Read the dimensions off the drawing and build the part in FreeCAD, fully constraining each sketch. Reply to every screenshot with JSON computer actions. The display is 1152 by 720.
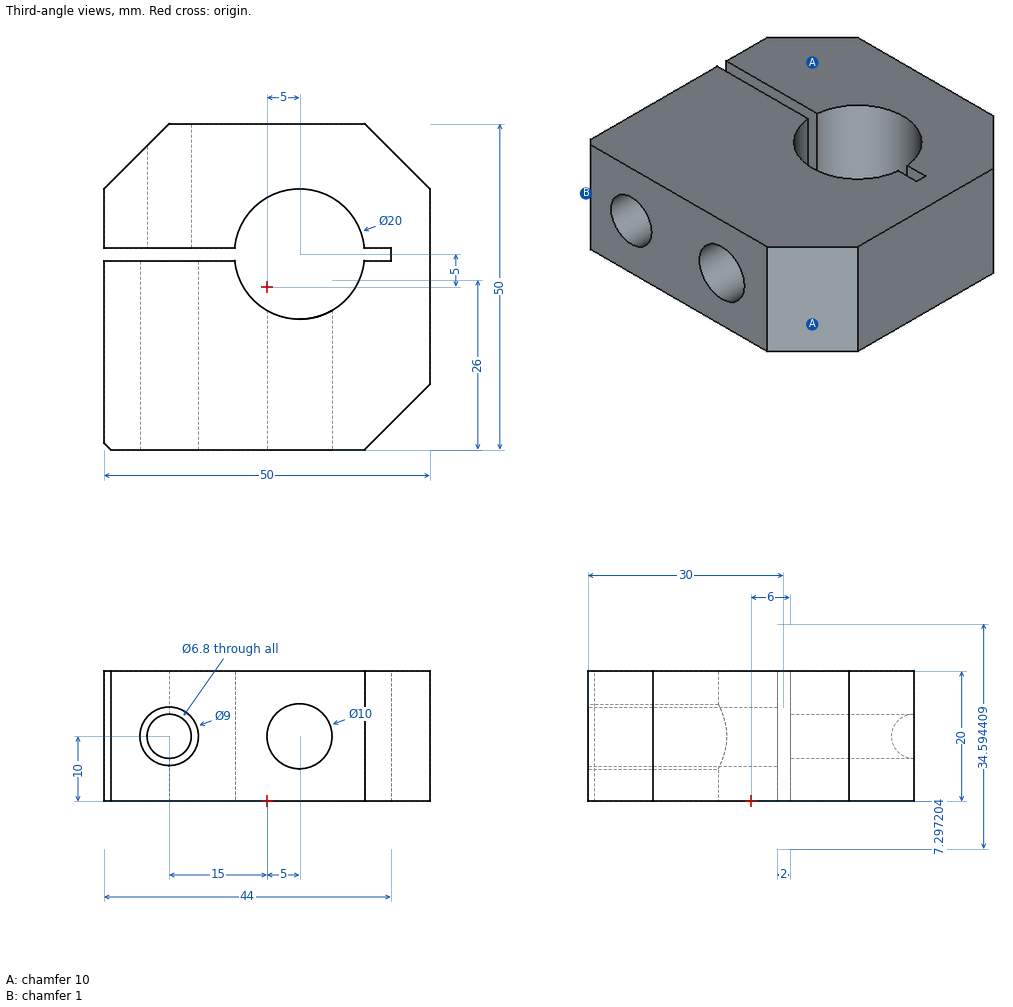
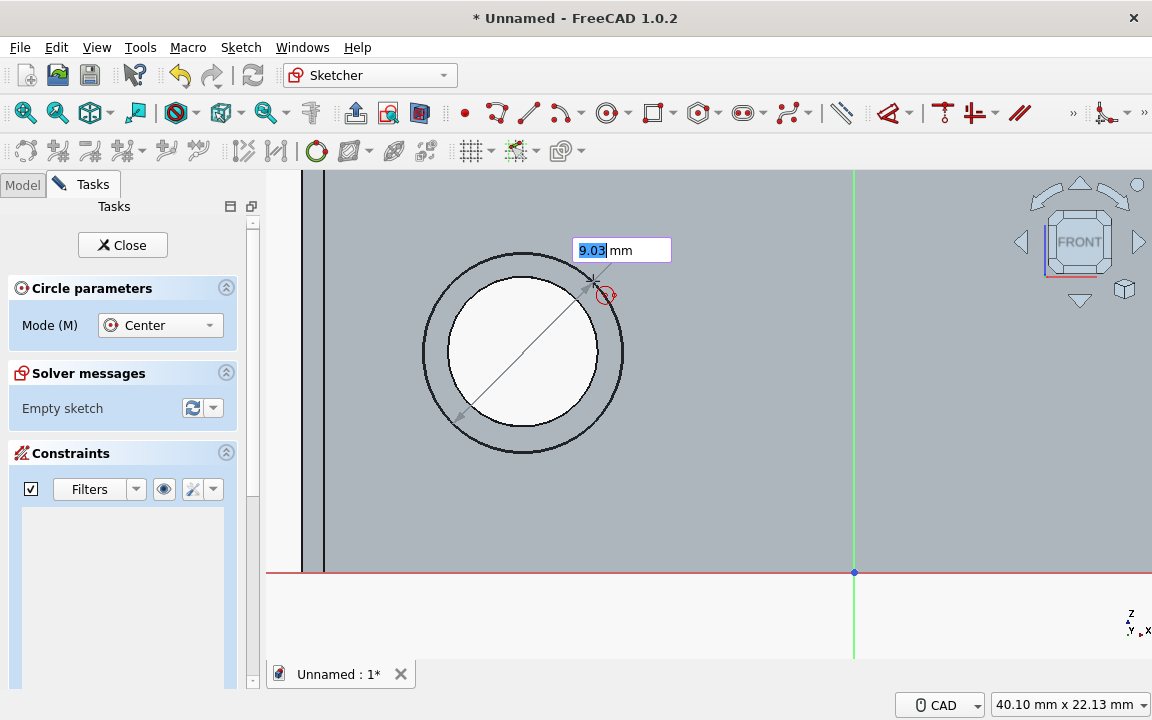
{"action": "type", "text": "9"}
{"action": "key", "text": "Return"}
{"action": "key", "text": "Escape"}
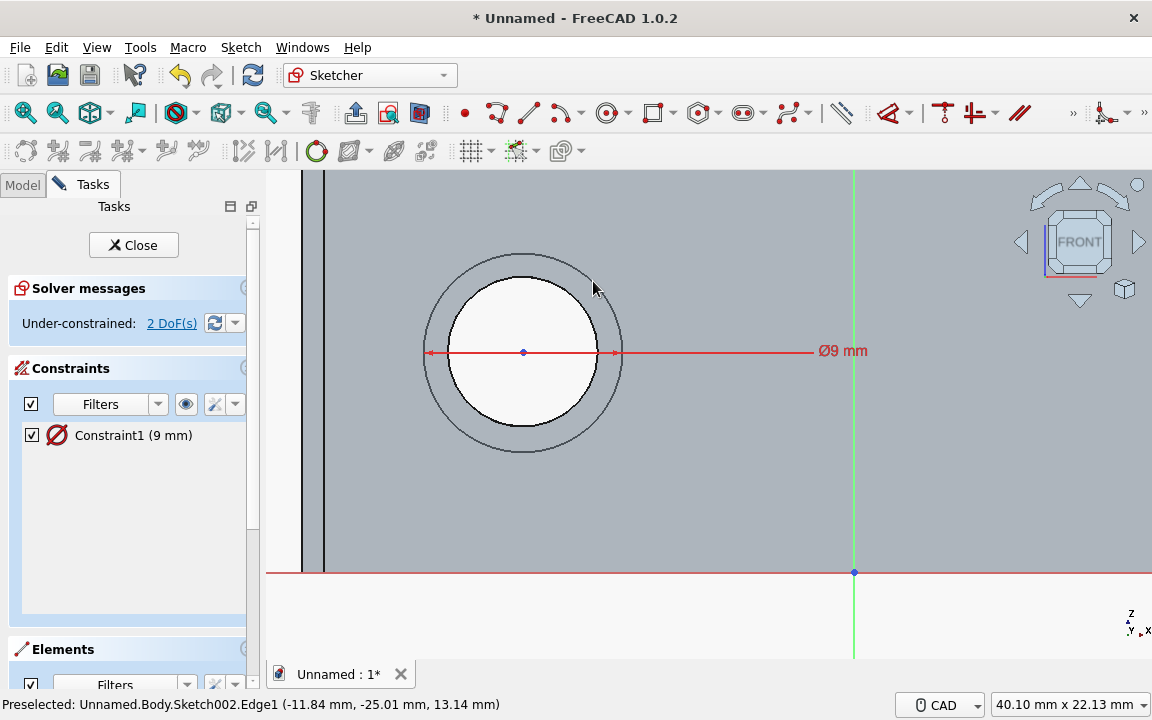
{"action": "left_click", "coordinate": [888, 114]}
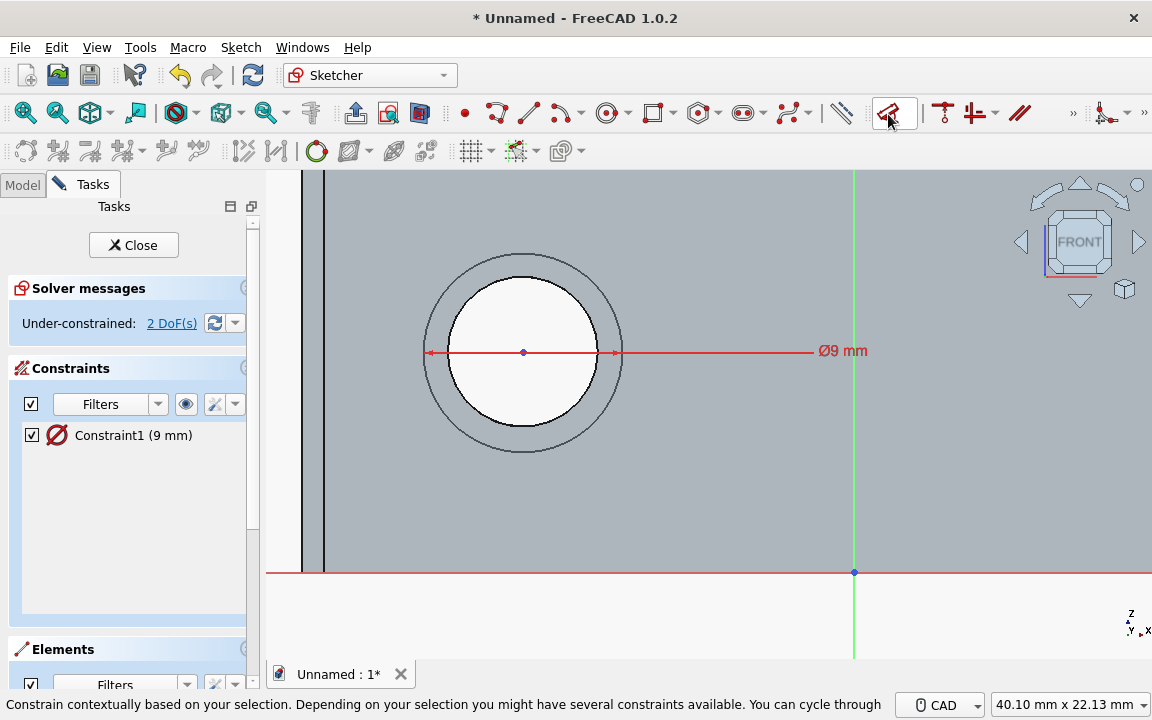
{"action": "left_click", "coordinate": [523, 353]}
{"action": "left_click", "coordinate": [689, 607]}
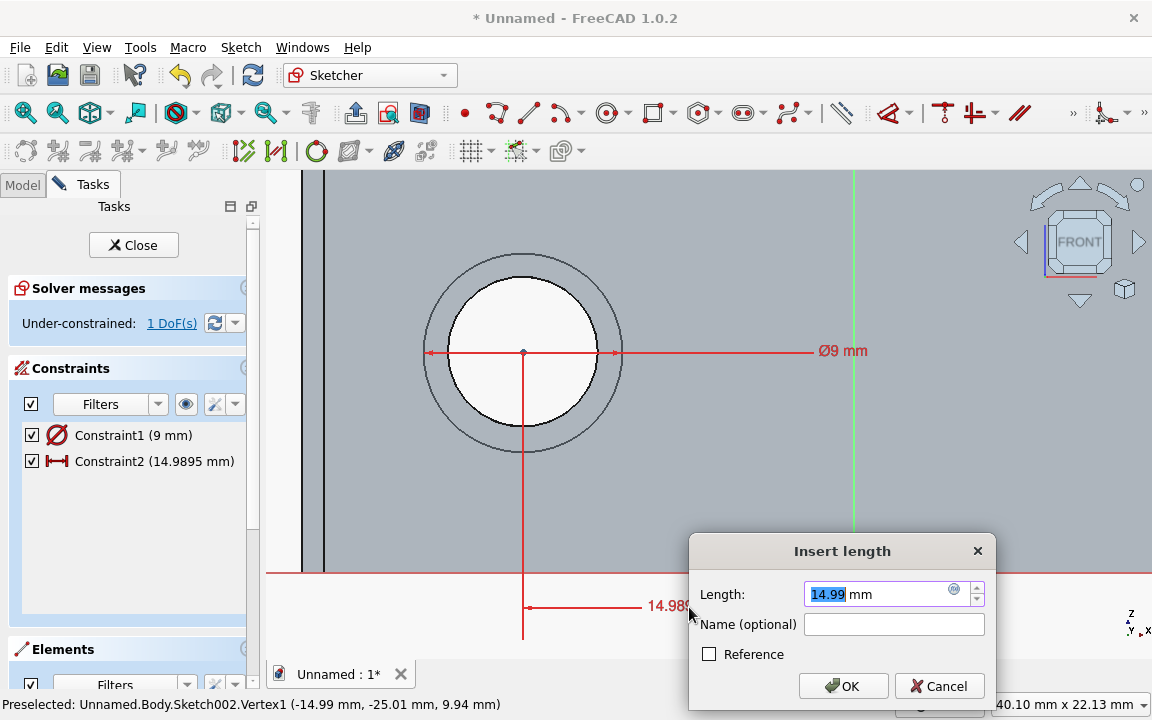
{"action": "type", "text": "15"}
{"action": "key", "text": "Return"}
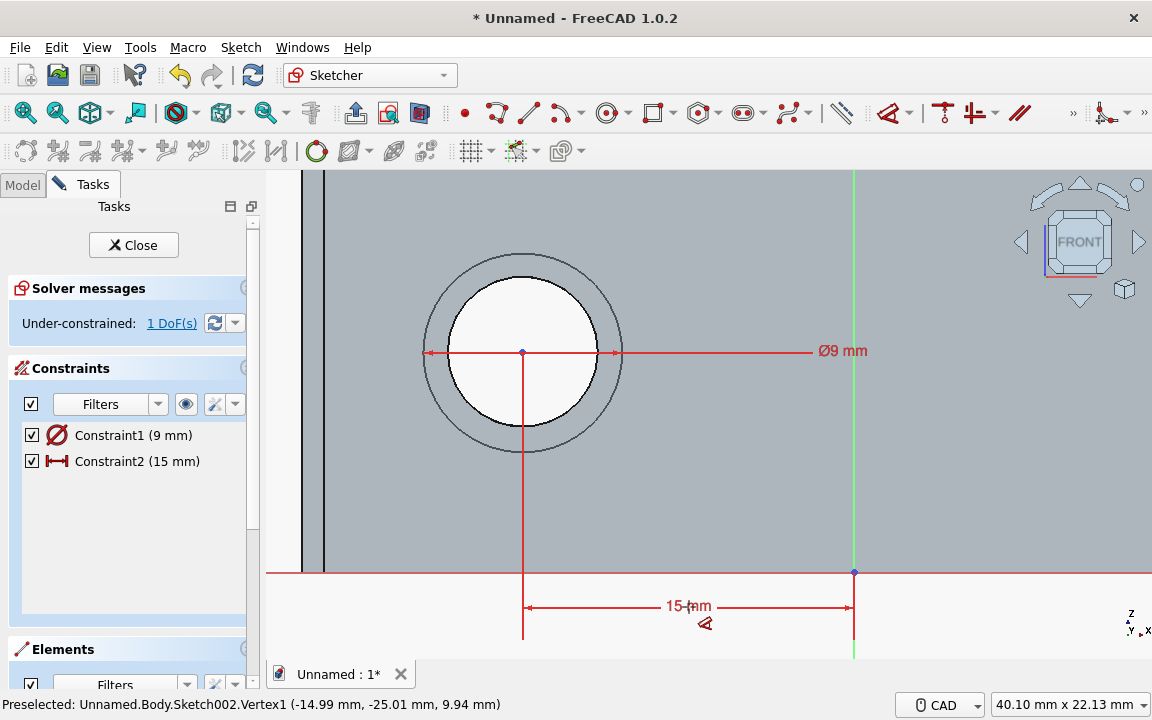
{"action": "left_click", "coordinate": [523, 353]}
{"action": "left_click", "coordinate": [888, 463]}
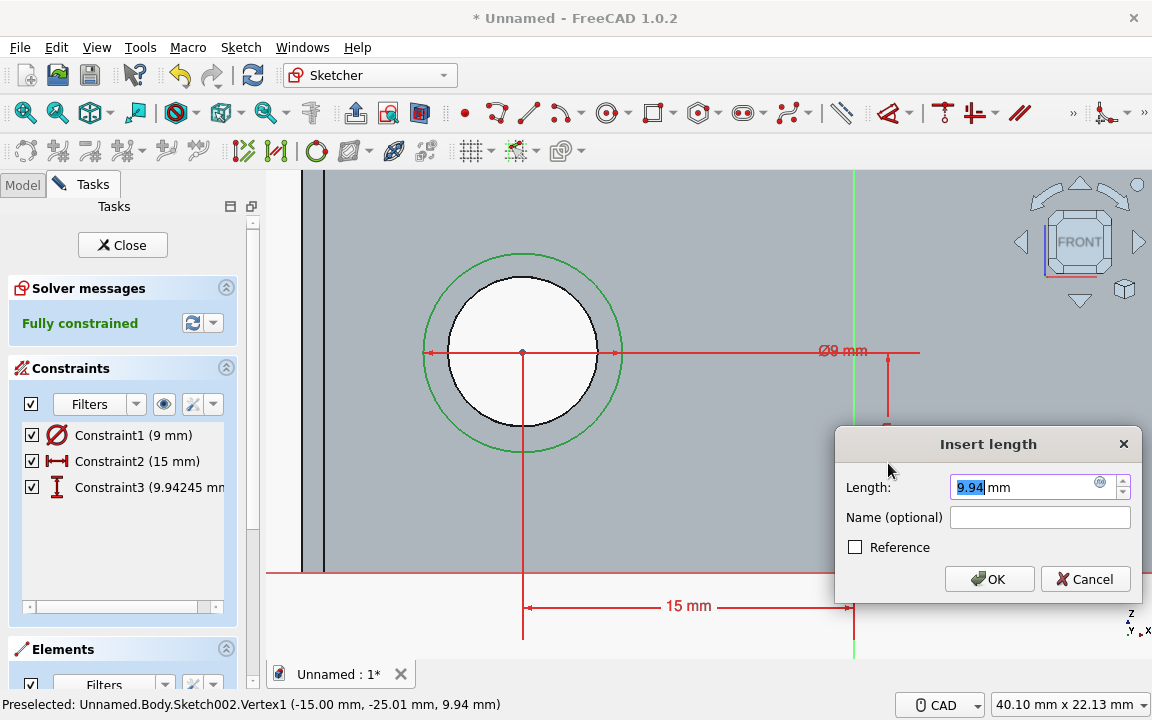
{"action": "type", "text": "10"}
{"action": "key", "text": "Return"}
{"action": "key", "text": "Escape"}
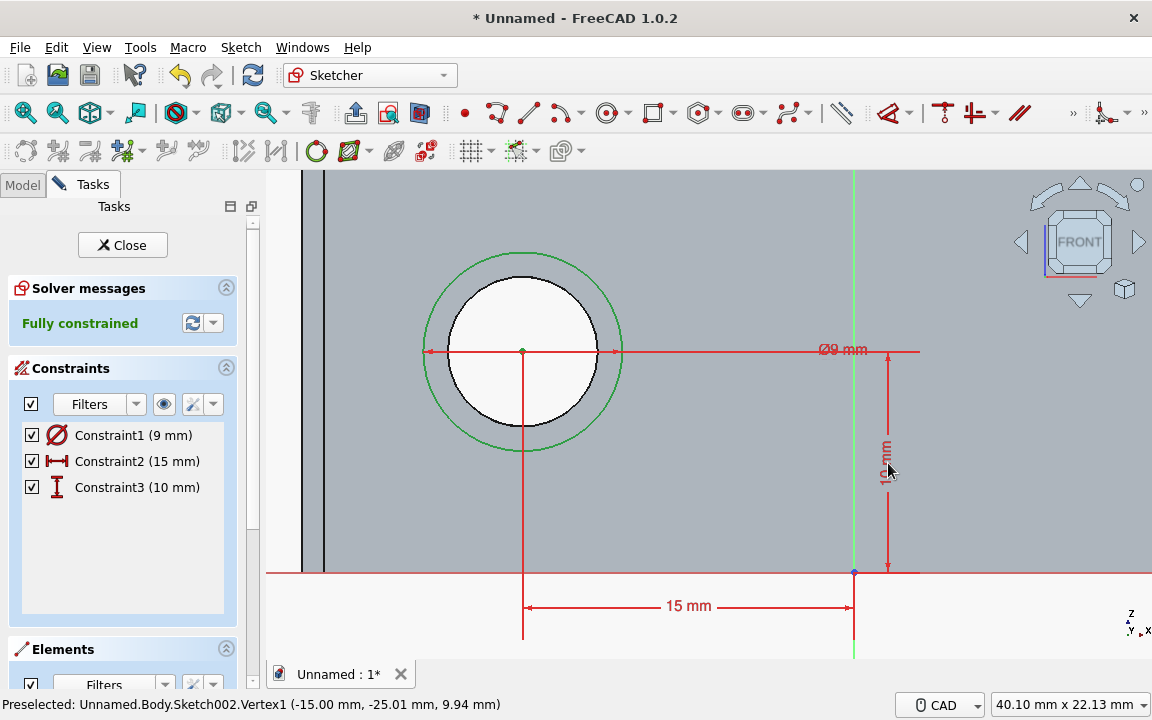
{"action": "left_click", "coordinate": [123, 245]}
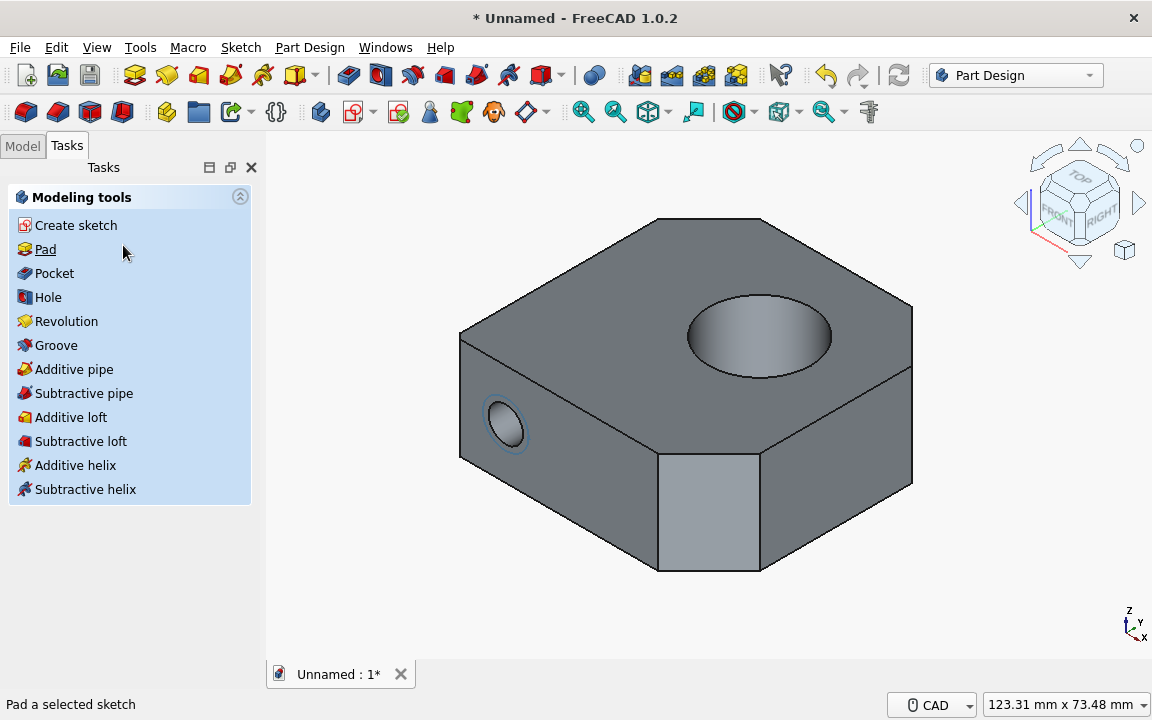
{"action": "left_click", "coordinate": [350, 76]}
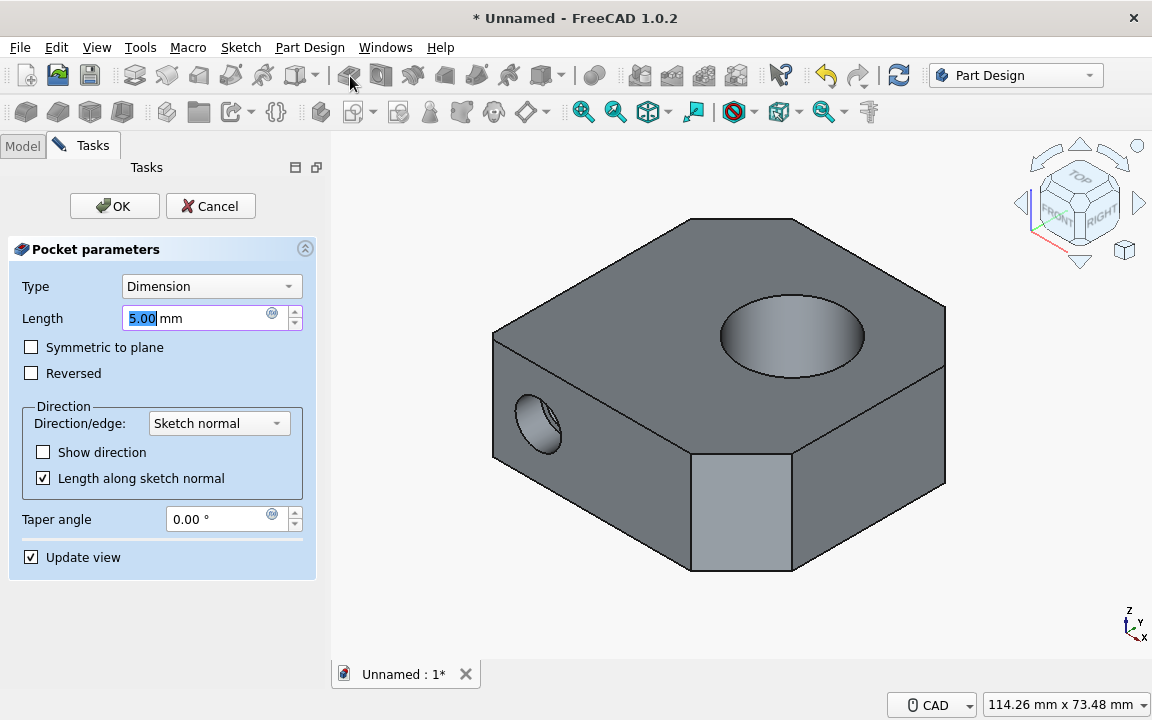
{"action": "type", "text": "30"}
{"action": "key", "text": "Tab"}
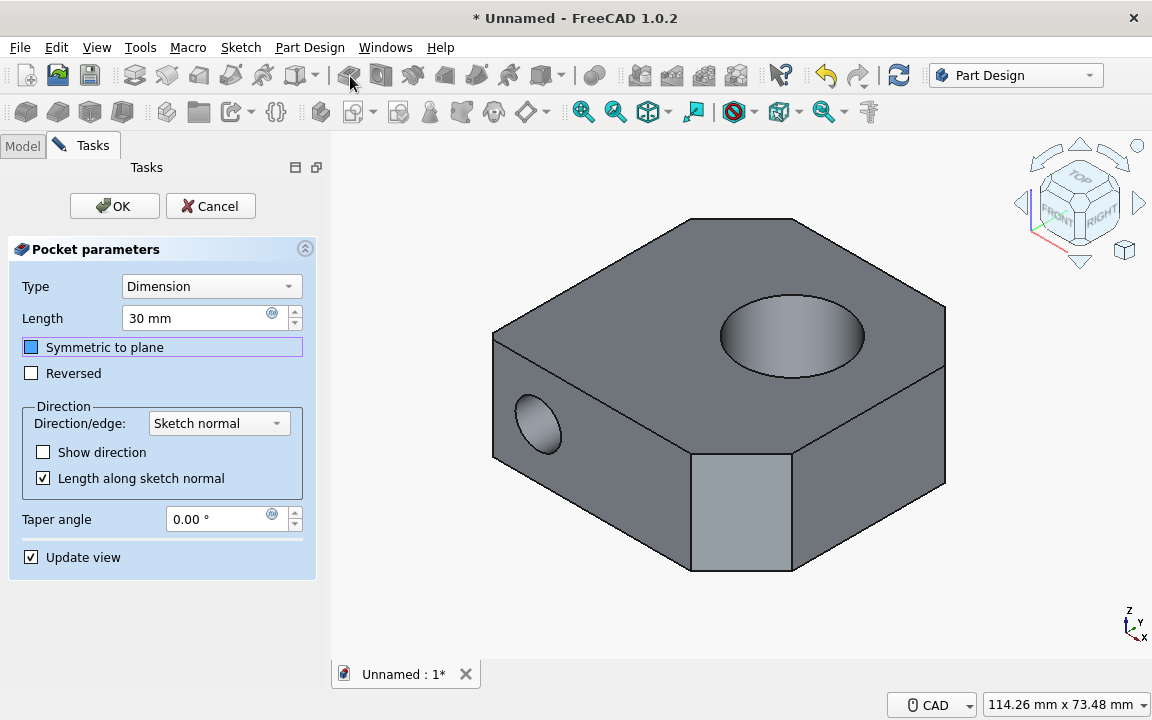
{"action": "left_click", "coordinate": [115, 206]}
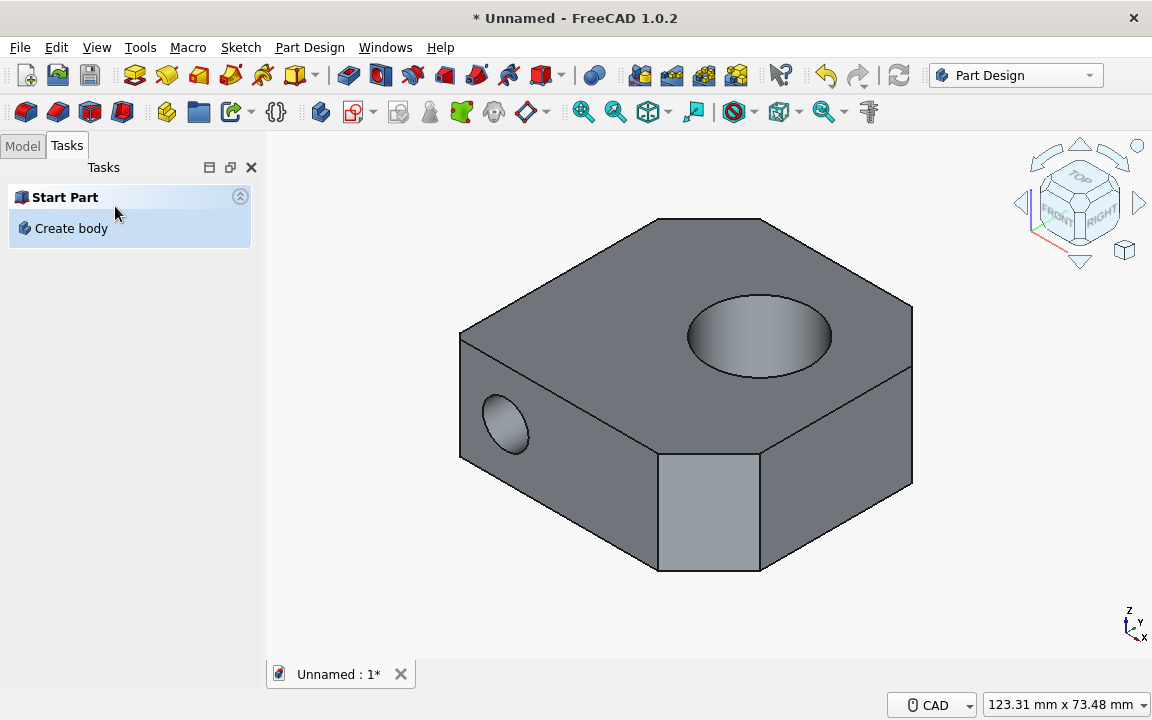
{"action": "key", "text": "6"}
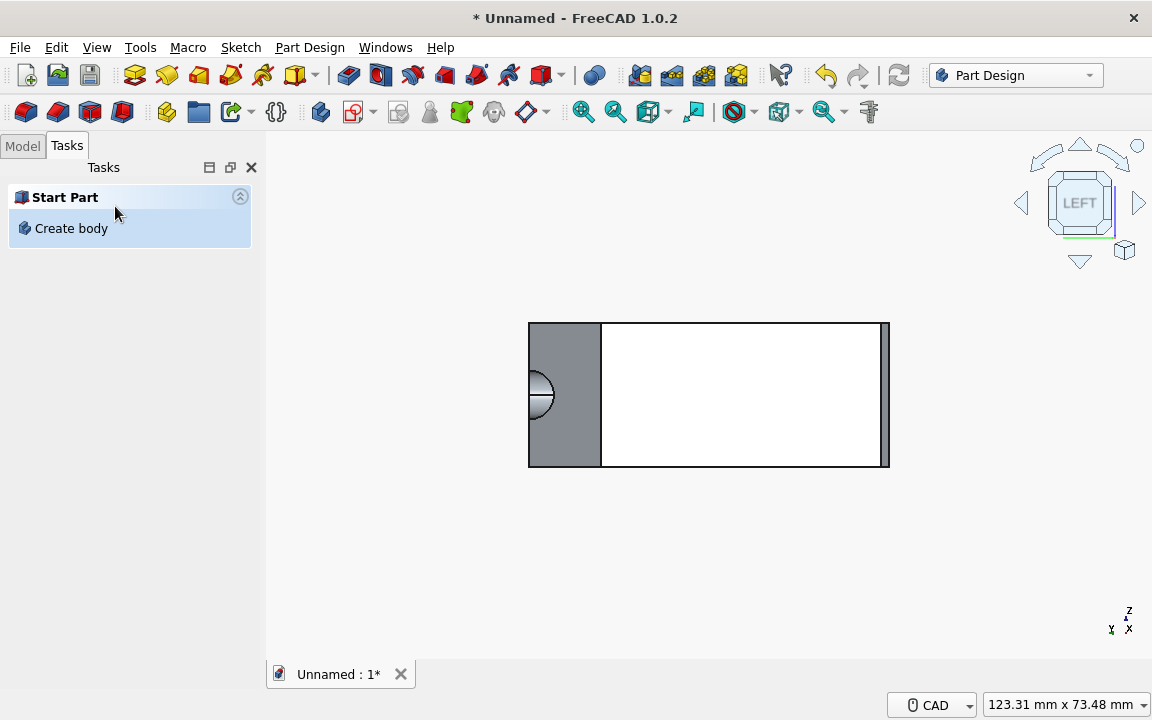
{"action": "left_click", "coordinate": [584, 112]}